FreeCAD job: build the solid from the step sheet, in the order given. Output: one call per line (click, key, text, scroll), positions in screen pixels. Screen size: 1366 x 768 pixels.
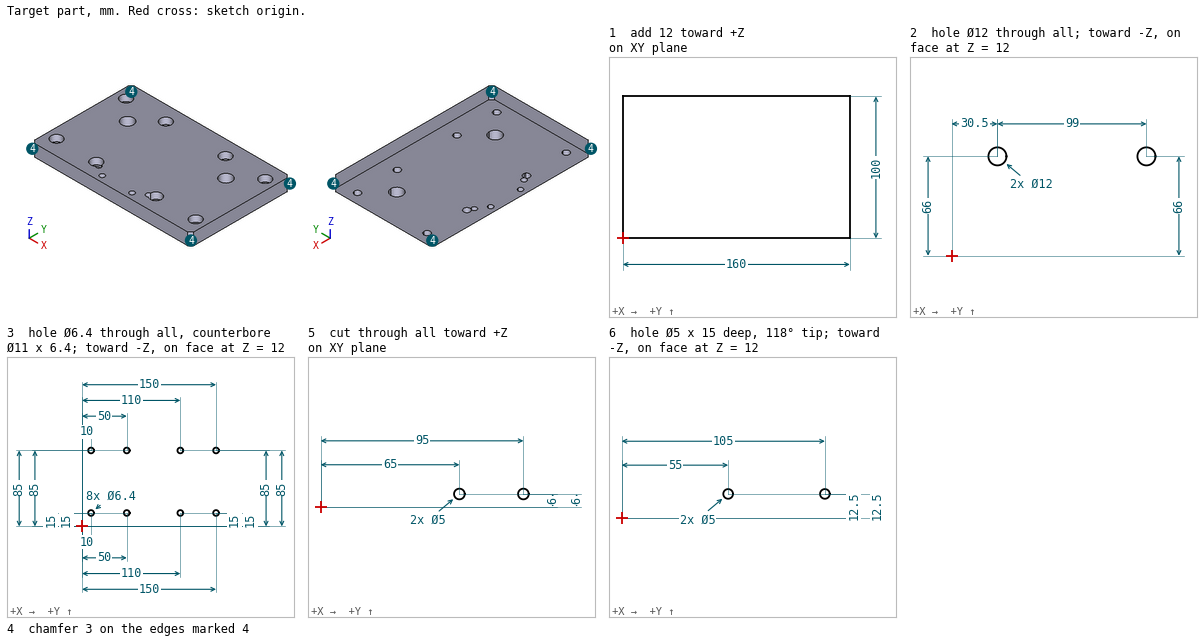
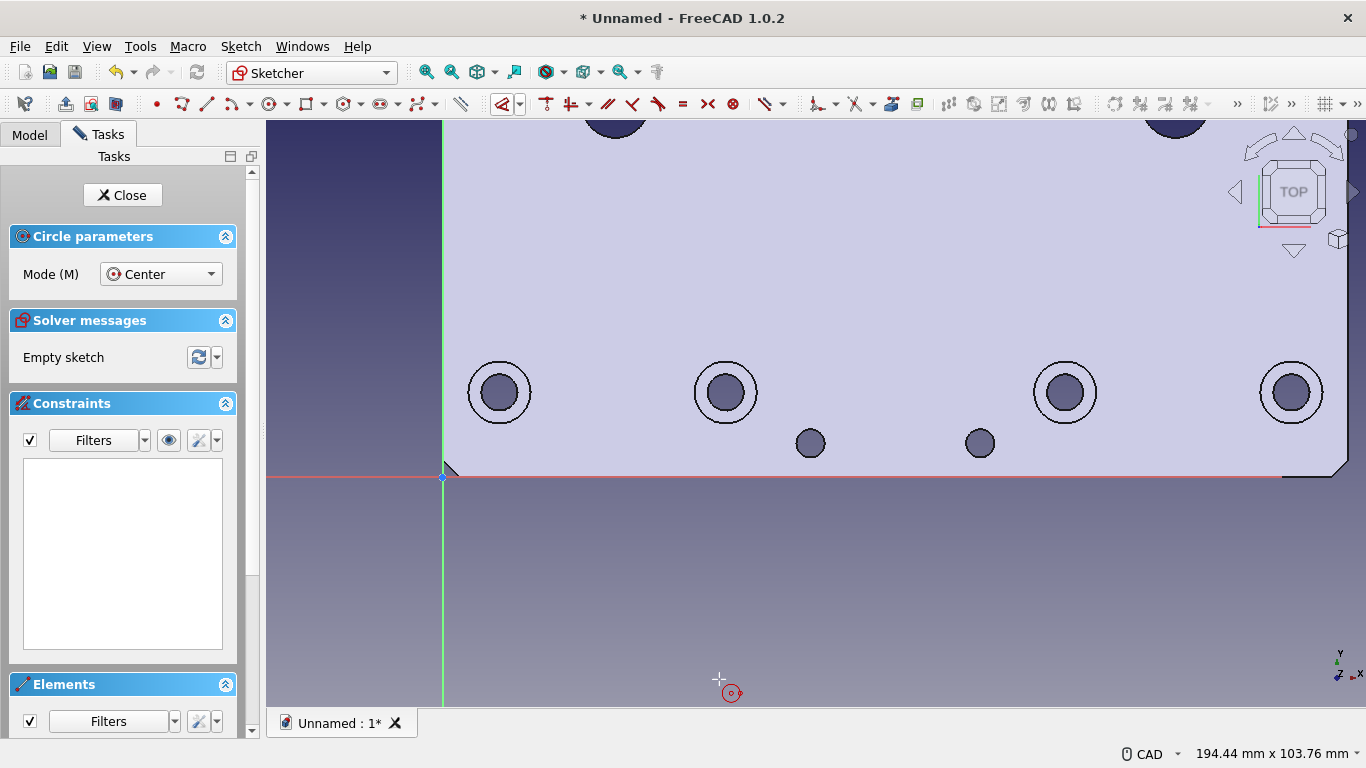
scroll(754, 407, up, 3)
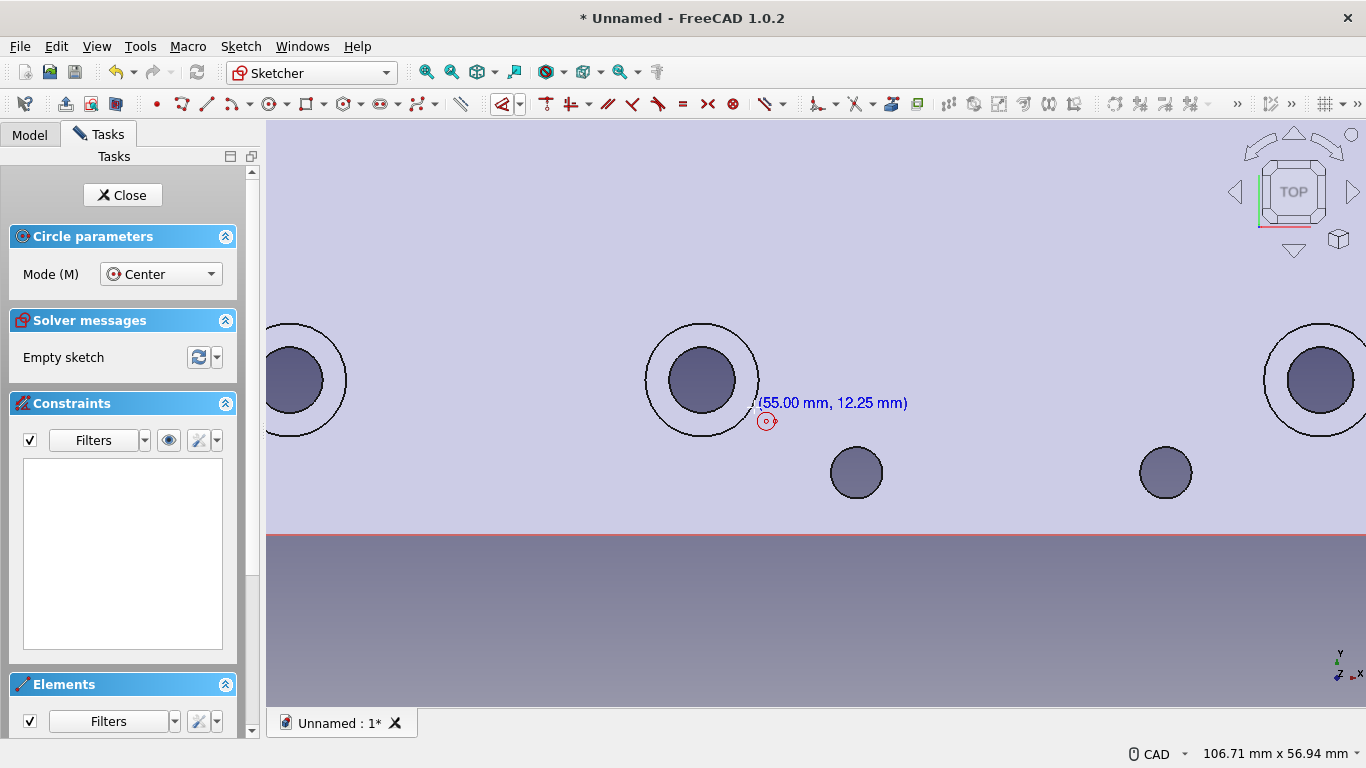
click(754, 406)
click(772, 388)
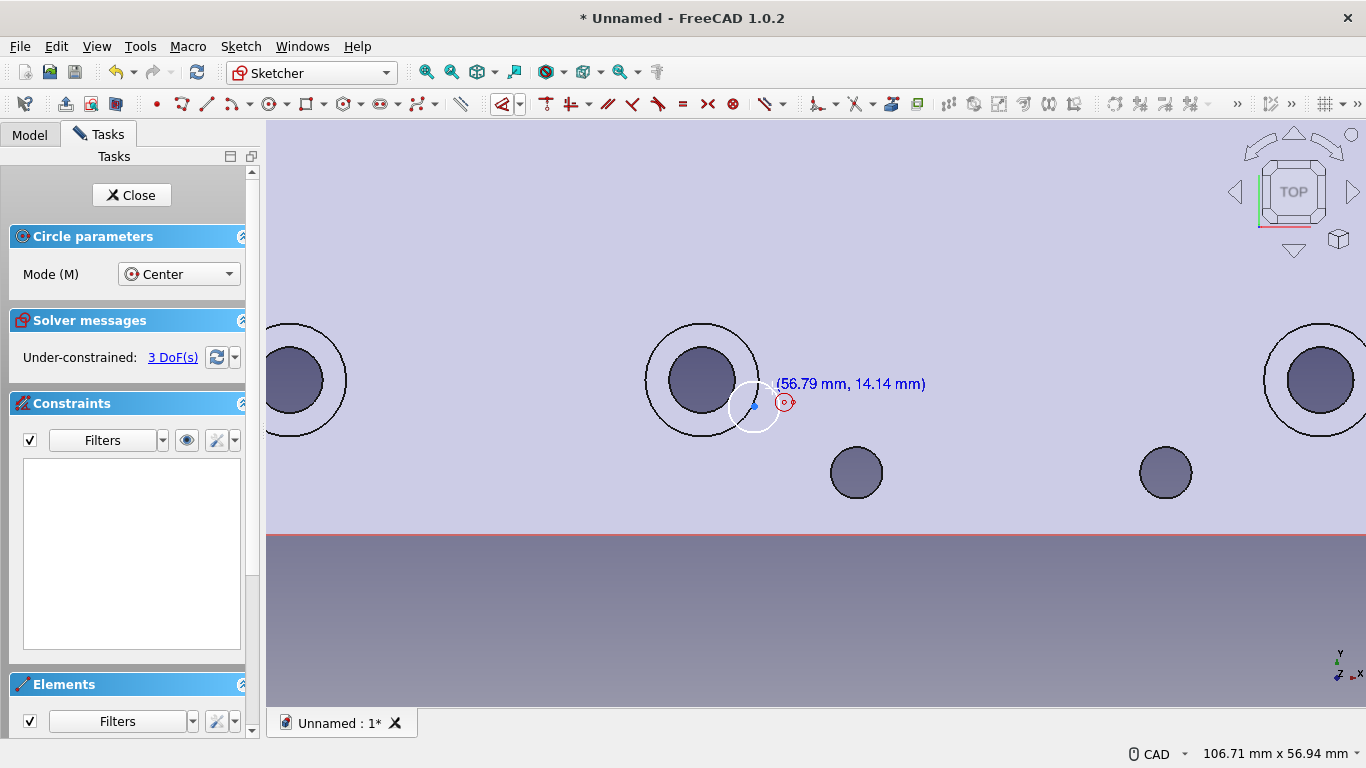
scroll(756, 360, down, 3)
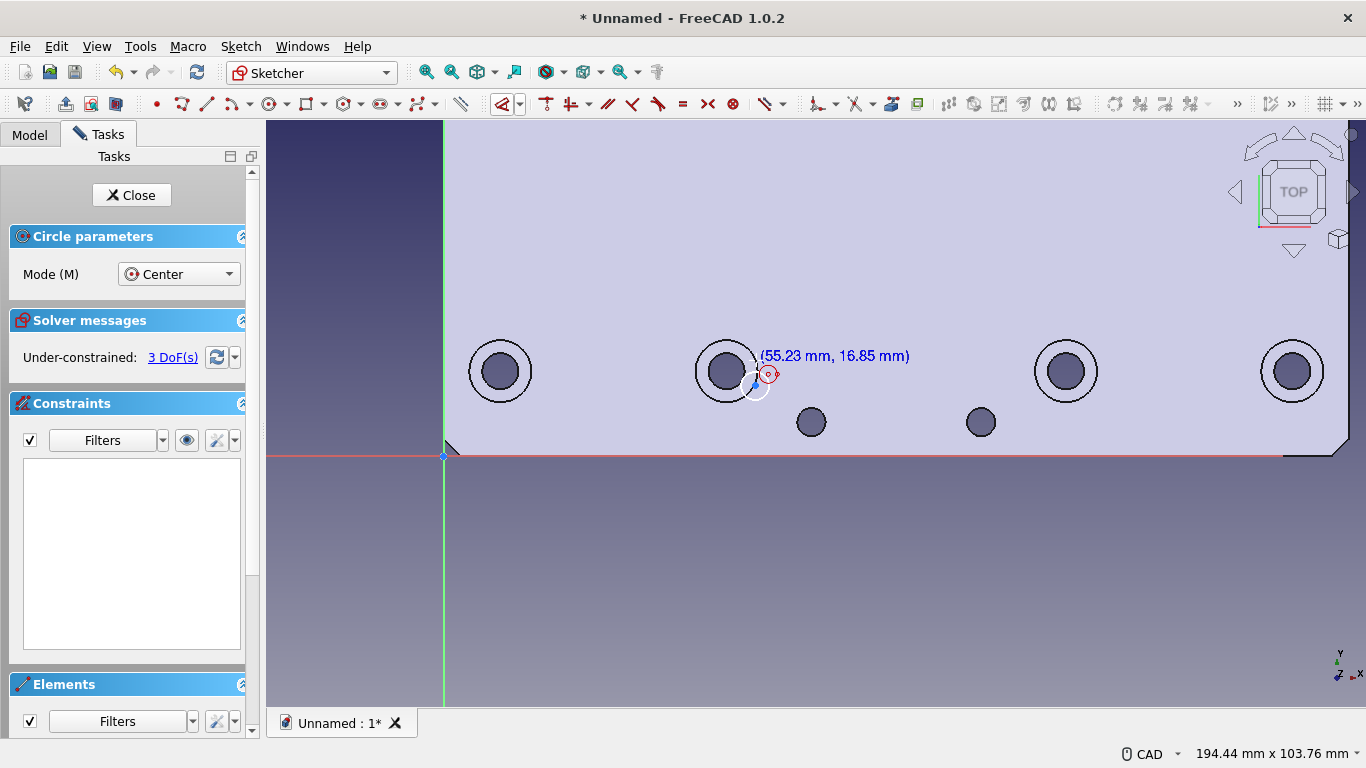
scroll(1038, 385, up, 3)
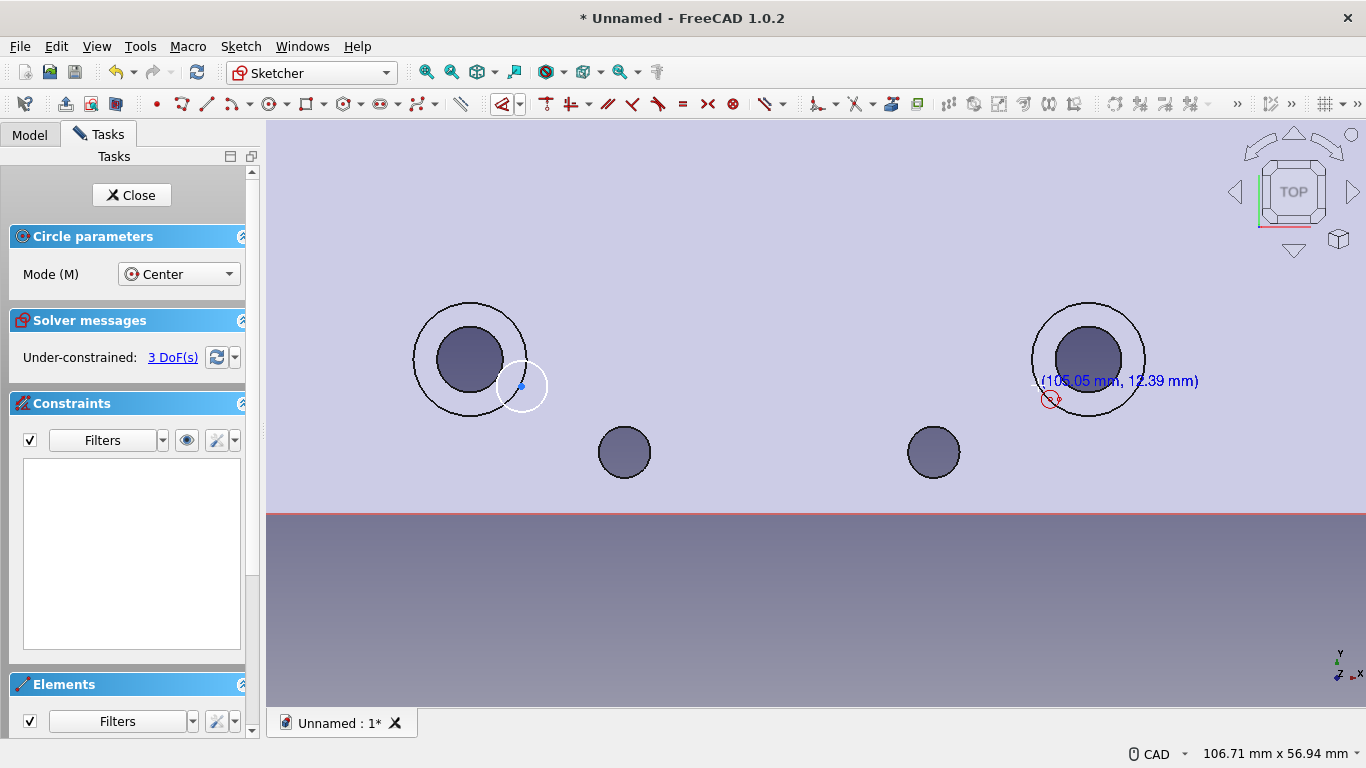
click(1037, 385)
click(1055, 367)
key(Escape)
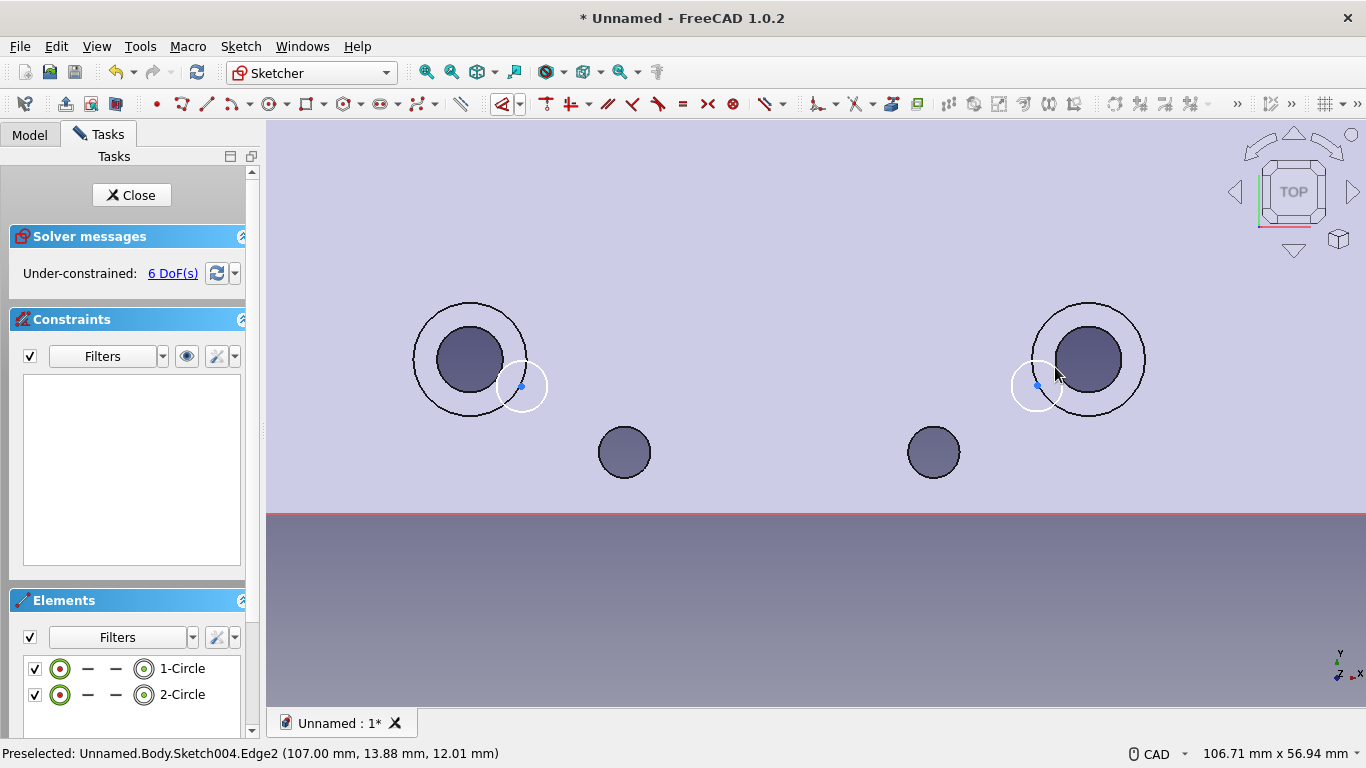
click(540, 368)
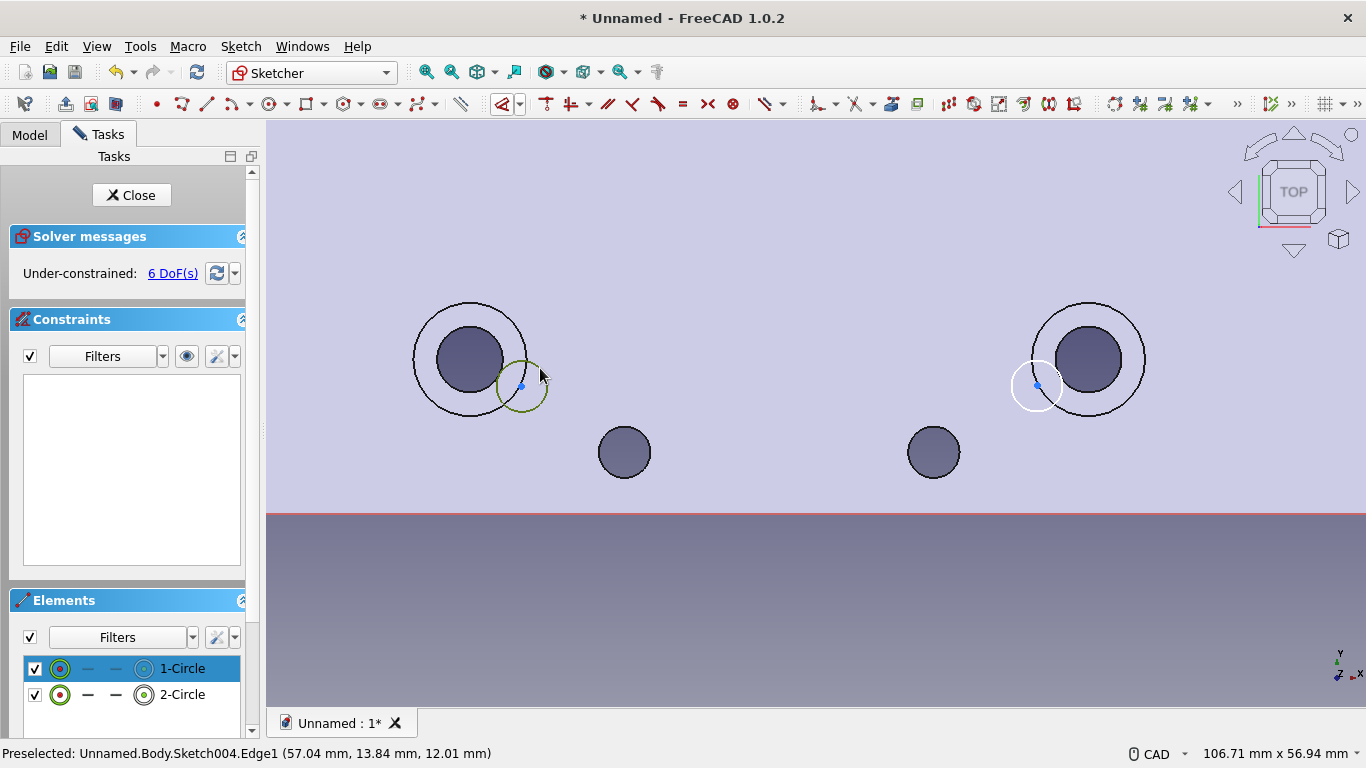
click(1055, 368)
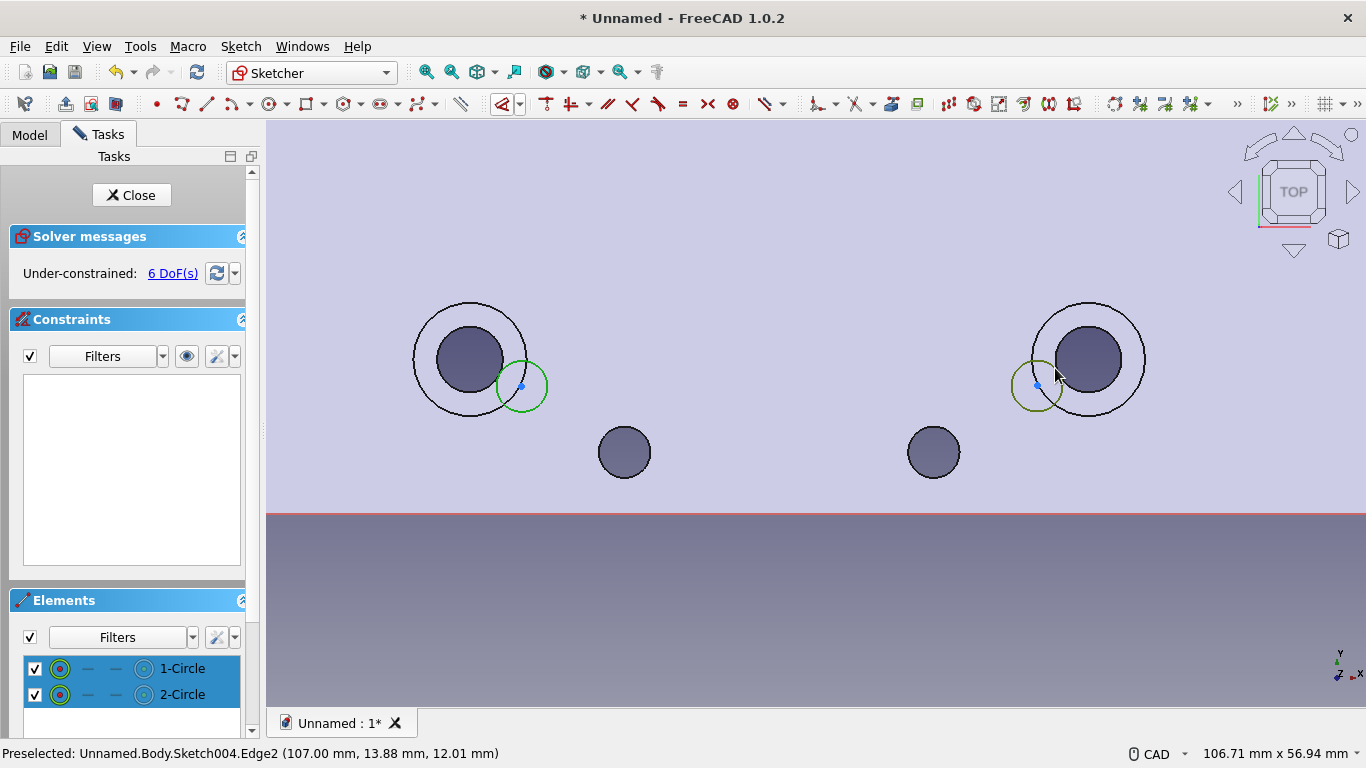
click(683, 104)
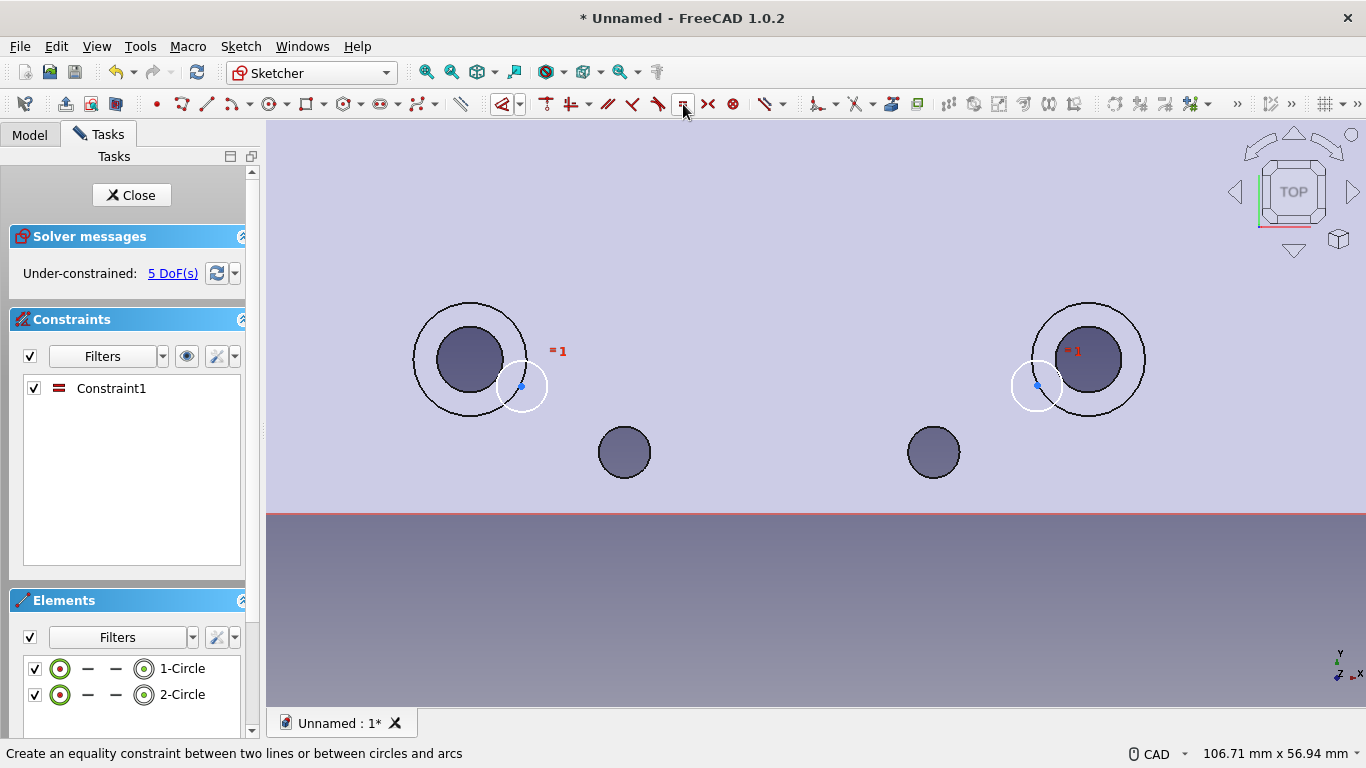
click(540, 368)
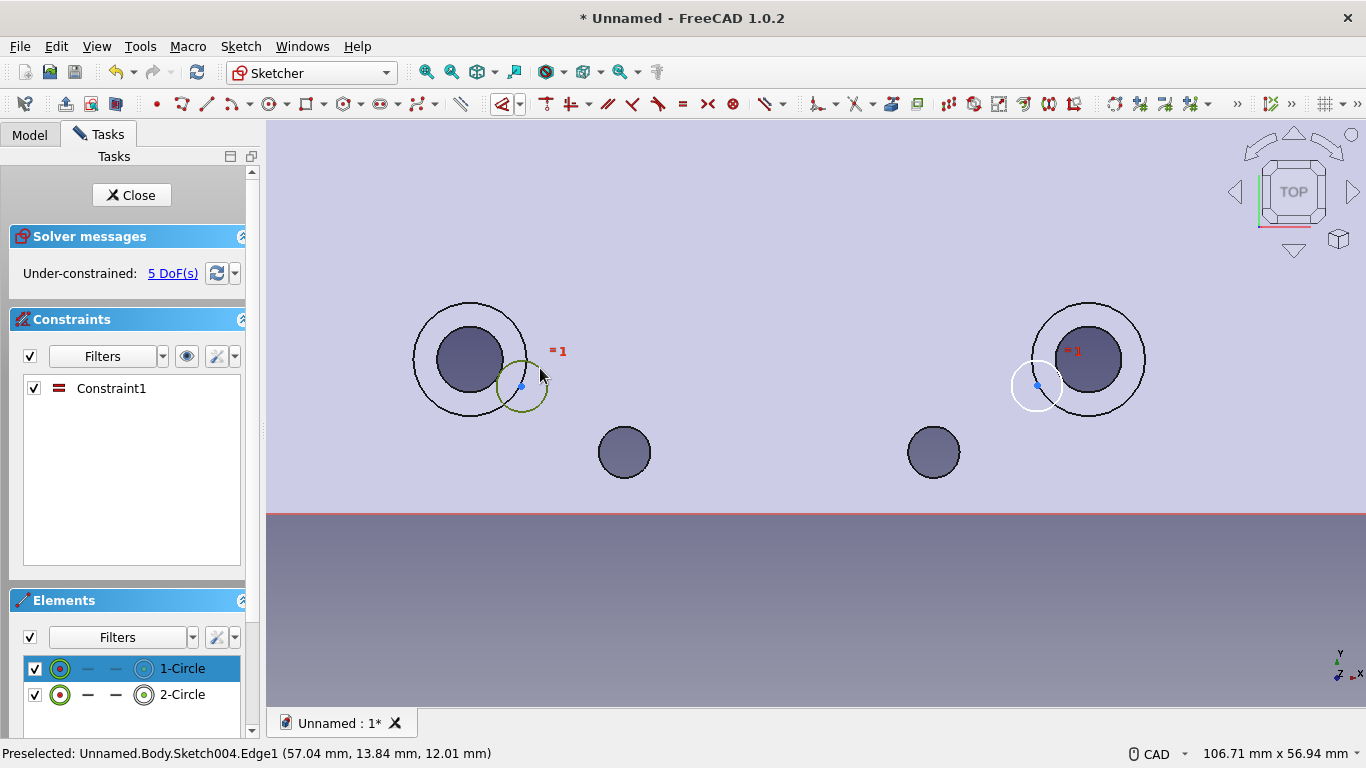
key(k)
key(o)